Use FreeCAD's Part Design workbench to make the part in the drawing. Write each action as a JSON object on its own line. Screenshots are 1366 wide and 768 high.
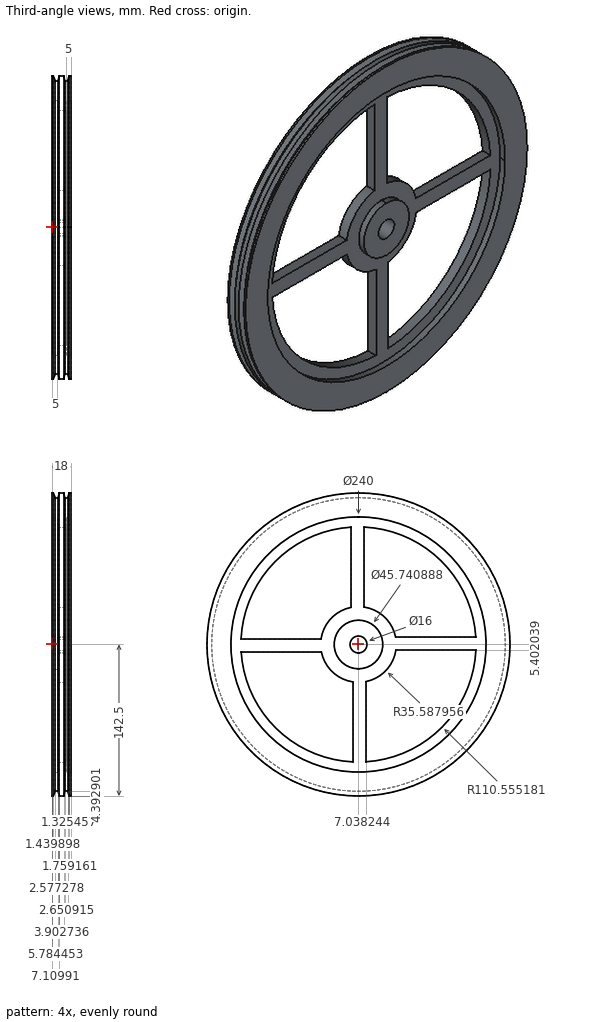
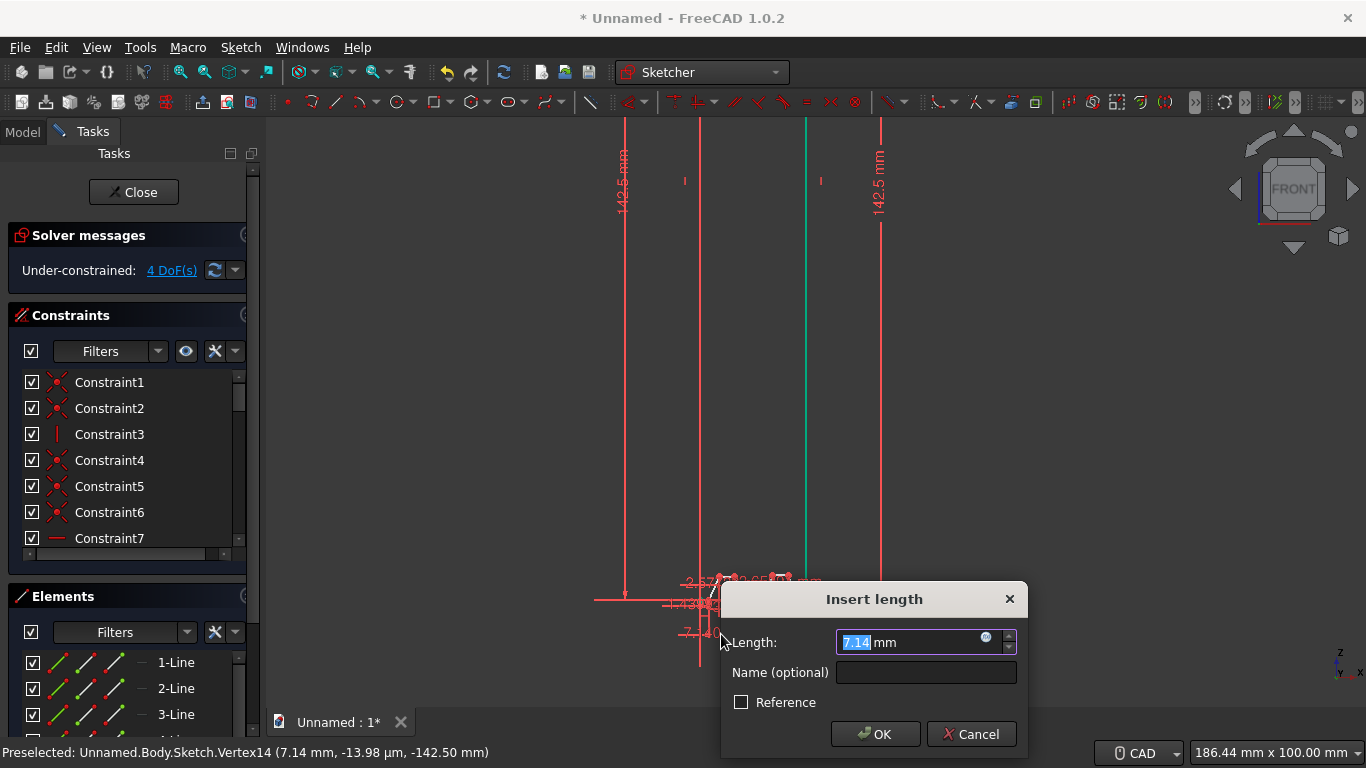
{"action": "type", "text": "7.10991"}
{"action": "key", "text": "Return"}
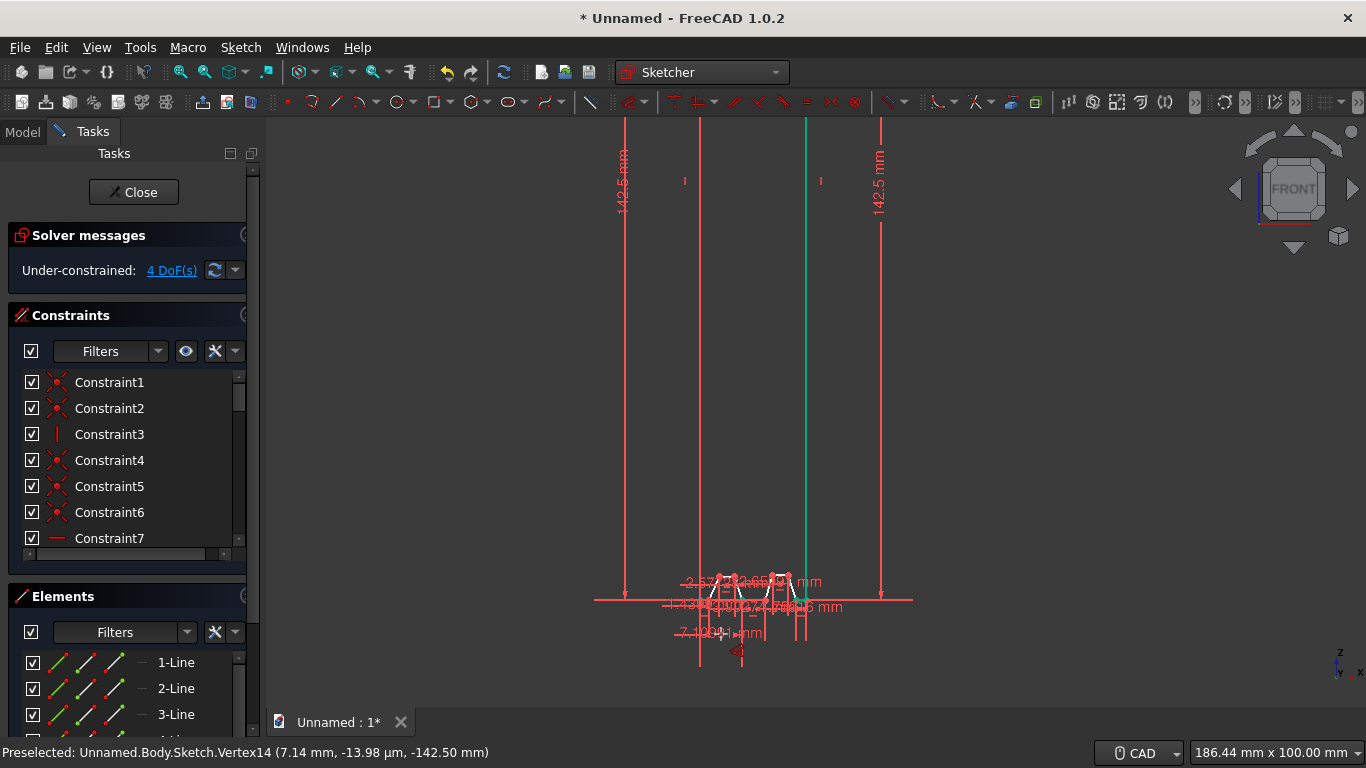
{"action": "left_click", "coordinate": [735, 577]}
{"action": "left_click", "coordinate": [717, 659]}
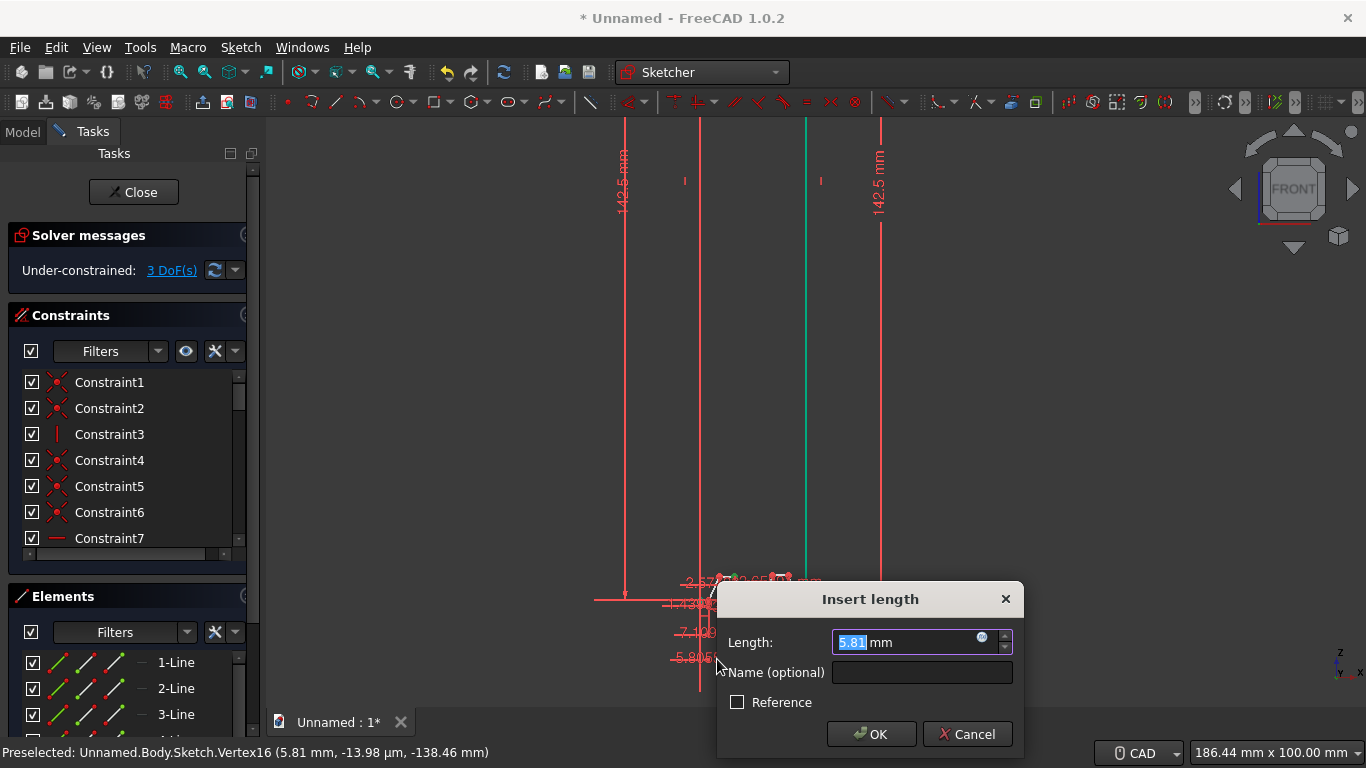
{"action": "type", "text": "5.784453"}
{"action": "key", "text": "Return"}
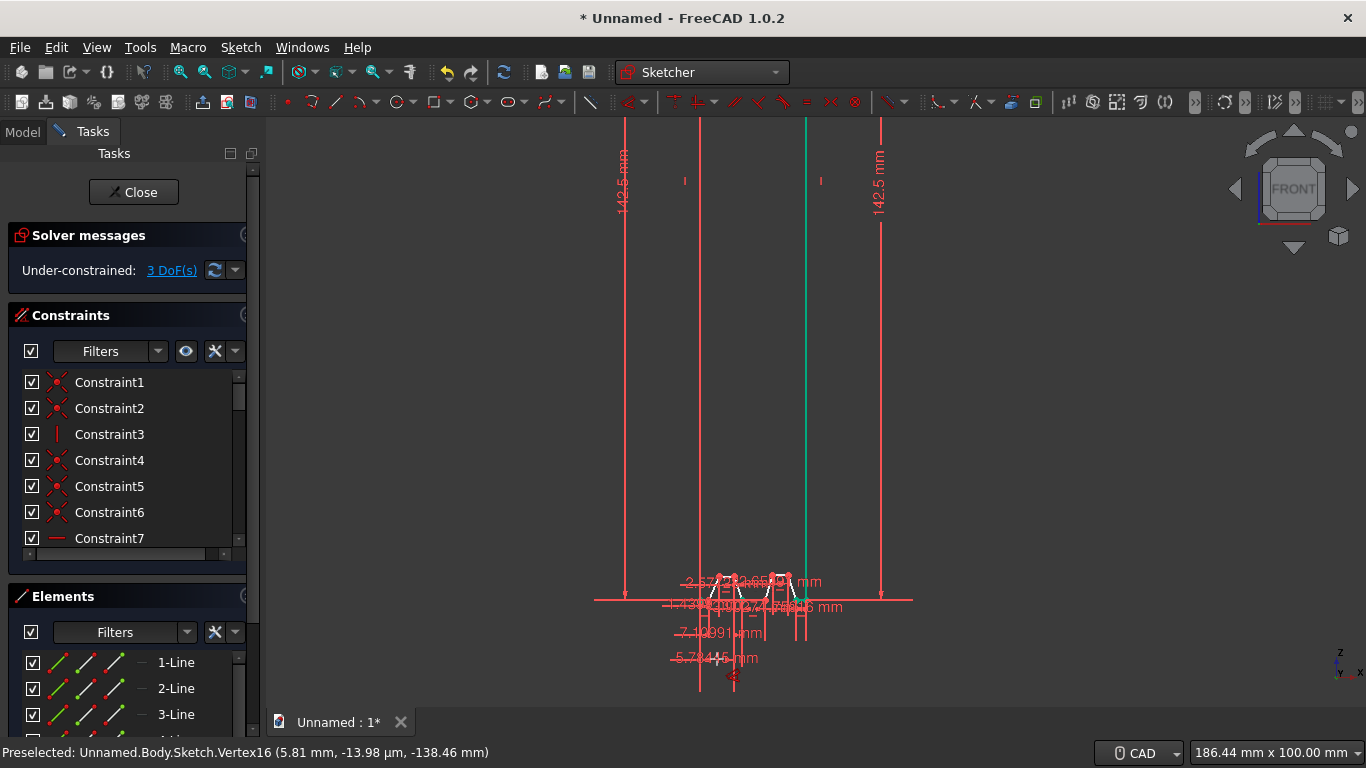
{"action": "scroll", "coordinate": [793, 590], "scroll_direction": "up", "scroll_amount": 9}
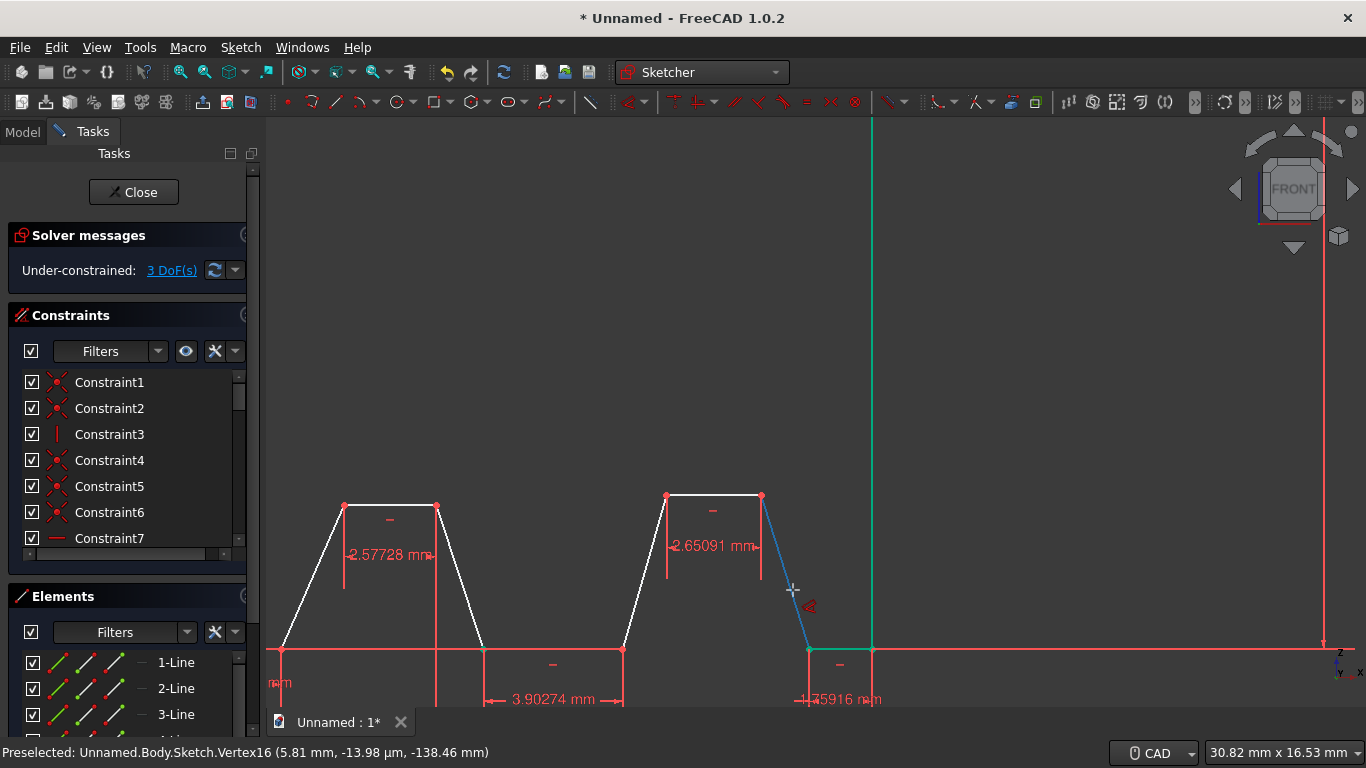
{"action": "left_click", "coordinate": [790, 588]}
{"action": "left_click", "coordinate": [785, 461]}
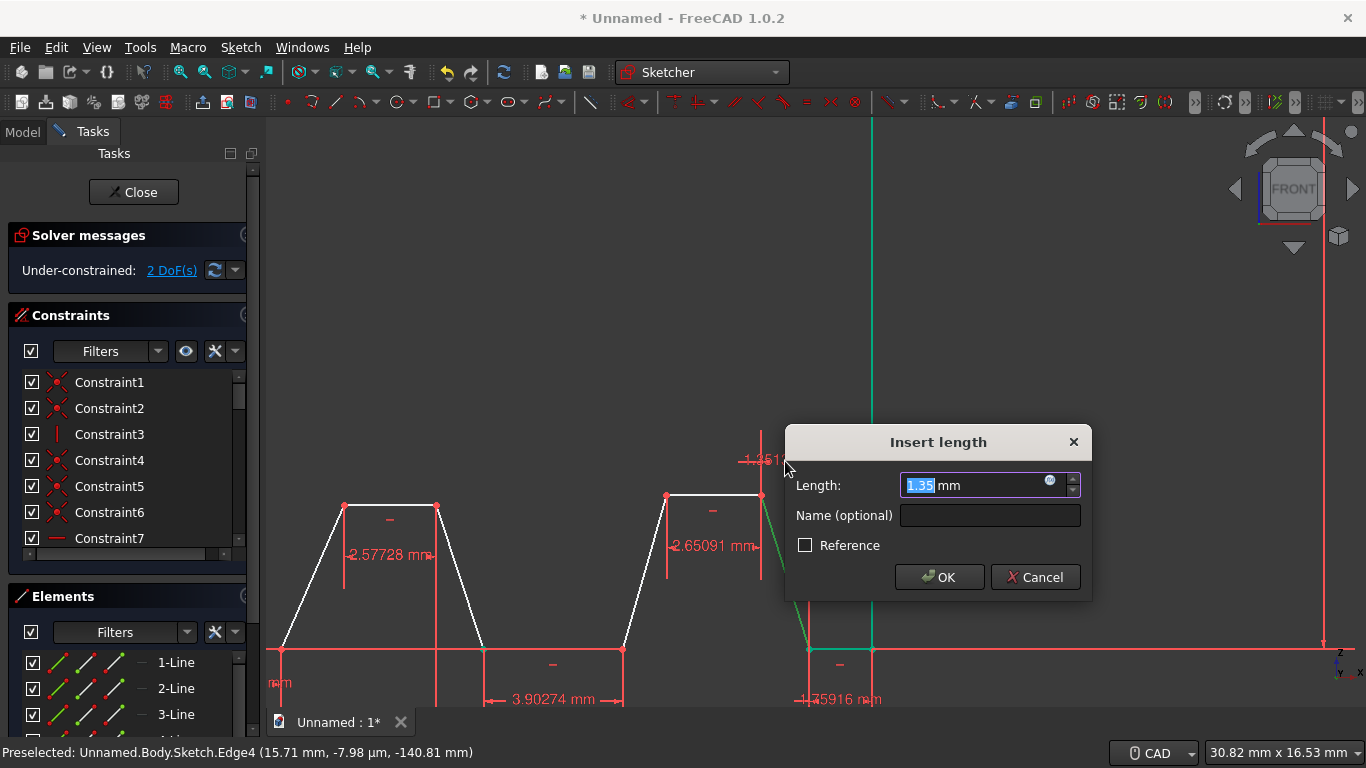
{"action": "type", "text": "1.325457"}
{"action": "key", "text": "Return"}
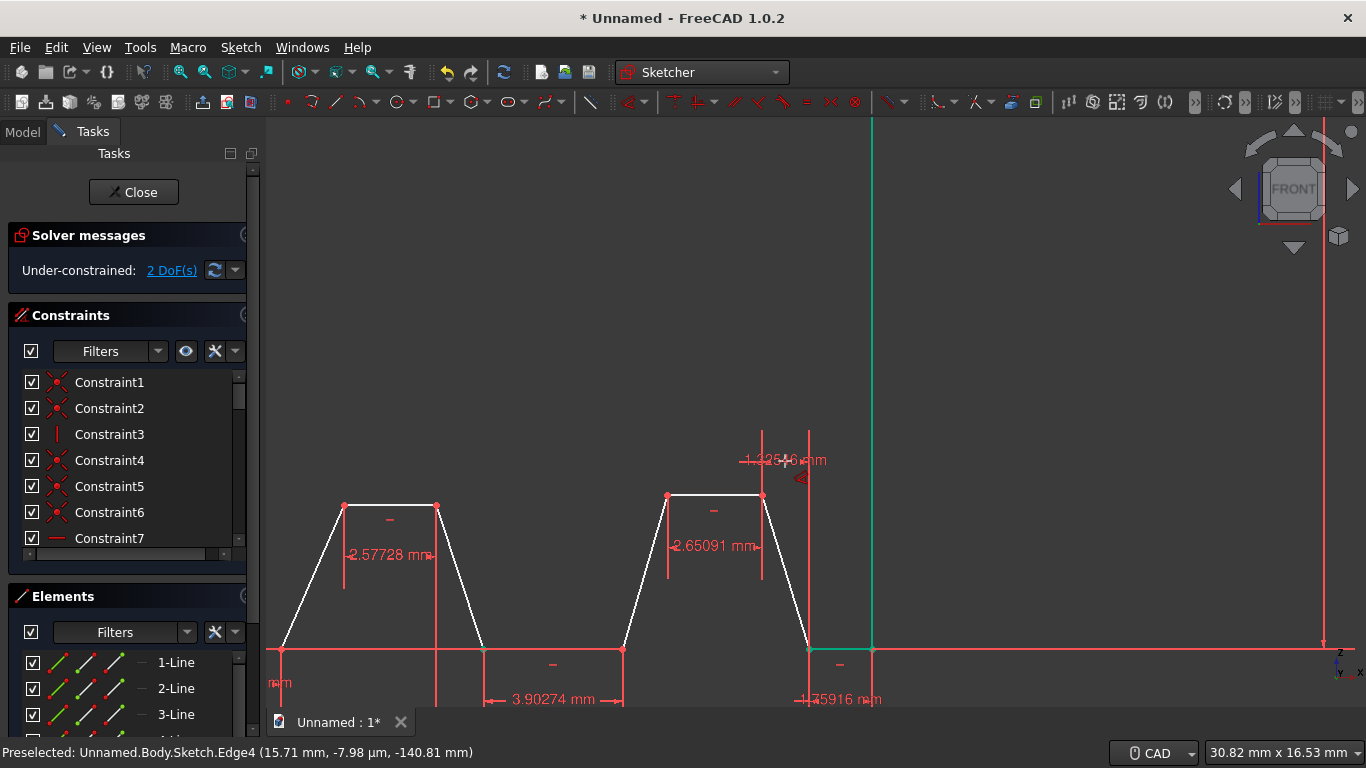
{"action": "scroll", "coordinate": [763, 597], "scroll_direction": "down", "scroll_amount": 13}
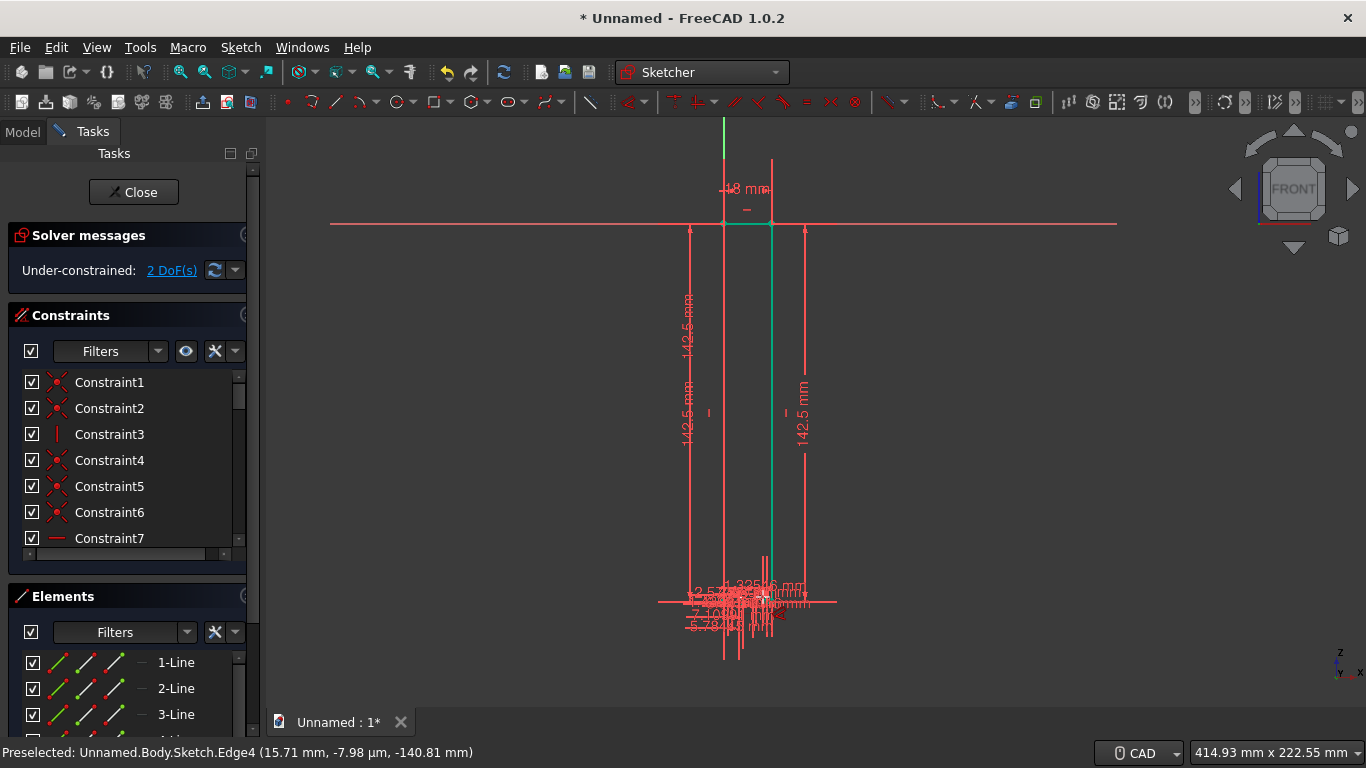
{"action": "scroll", "coordinate": [766, 598], "scroll_direction": "up", "scroll_amount": 7}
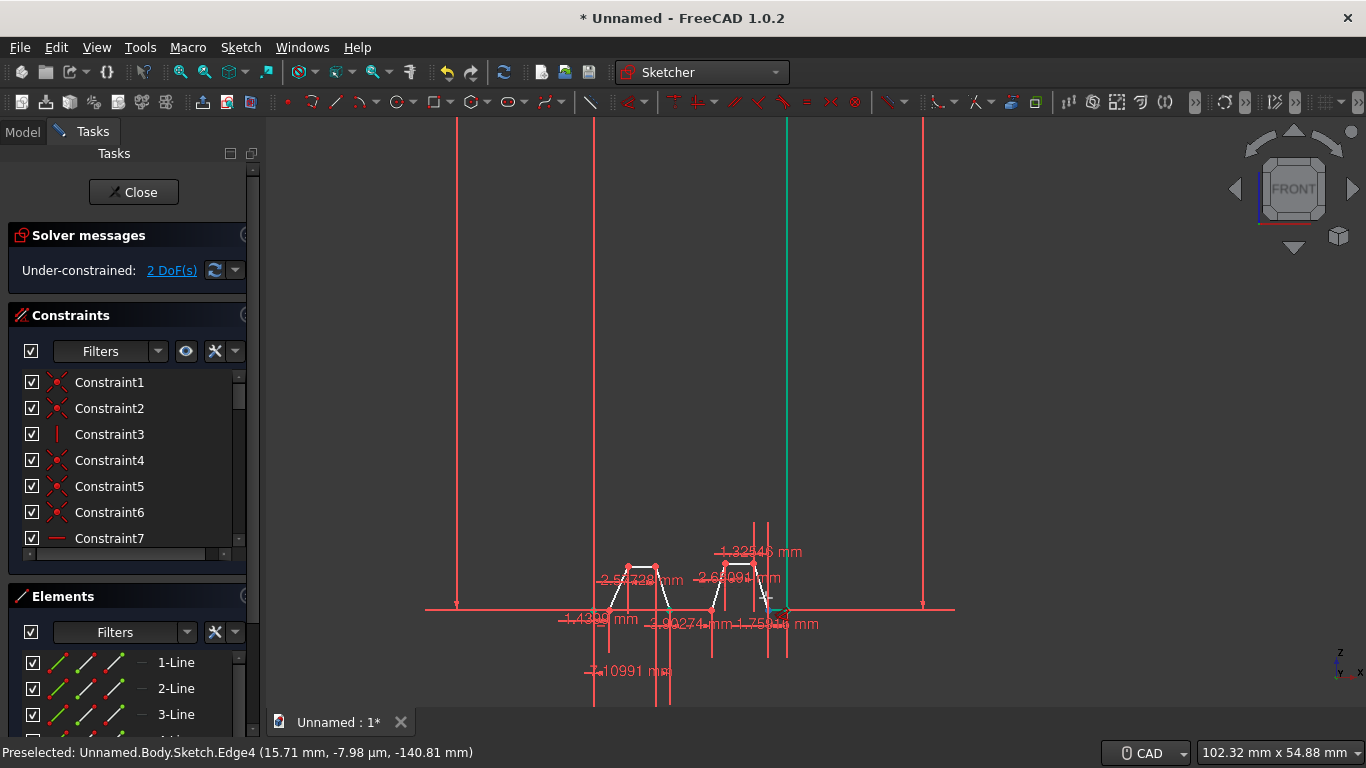
{"action": "left_click", "coordinate": [764, 596]}
{"action": "left_click", "coordinate": [802, 603]}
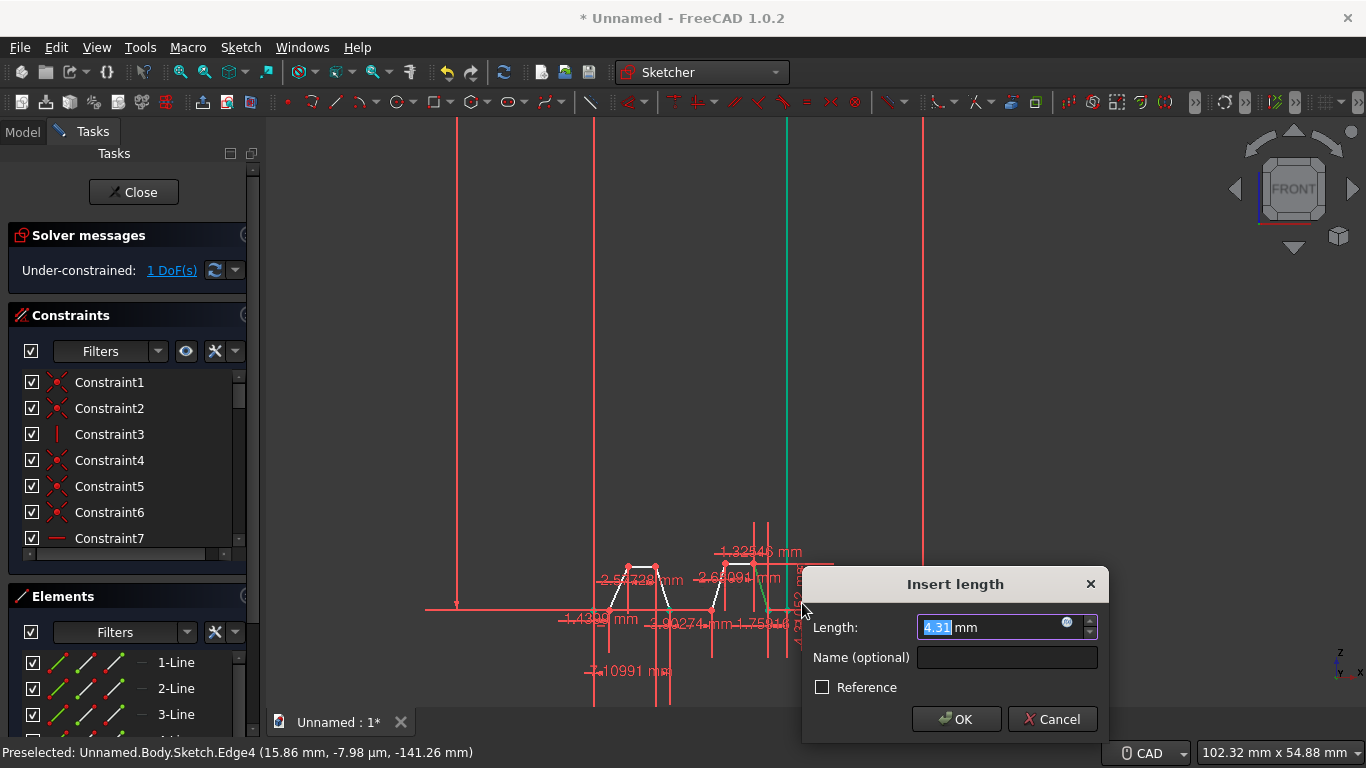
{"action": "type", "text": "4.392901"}
{"action": "key", "text": "Return"}